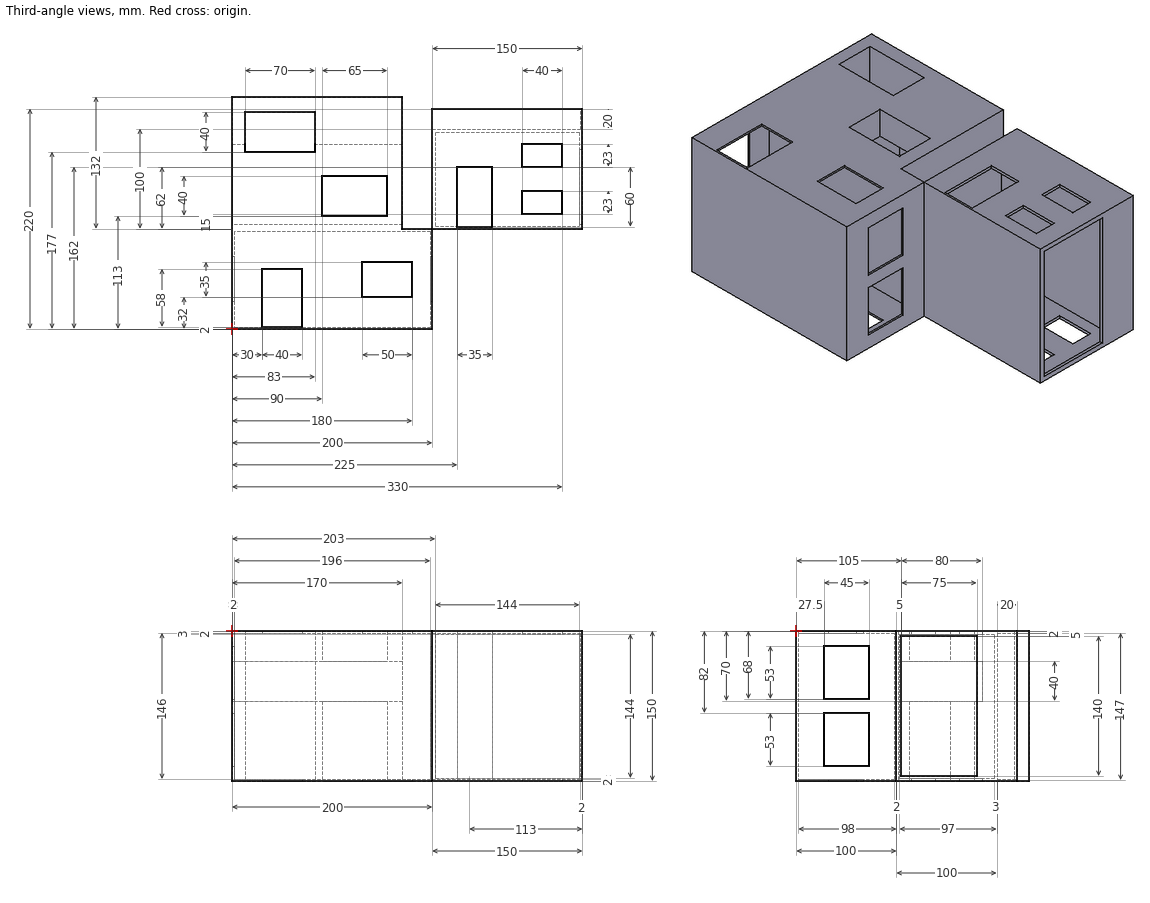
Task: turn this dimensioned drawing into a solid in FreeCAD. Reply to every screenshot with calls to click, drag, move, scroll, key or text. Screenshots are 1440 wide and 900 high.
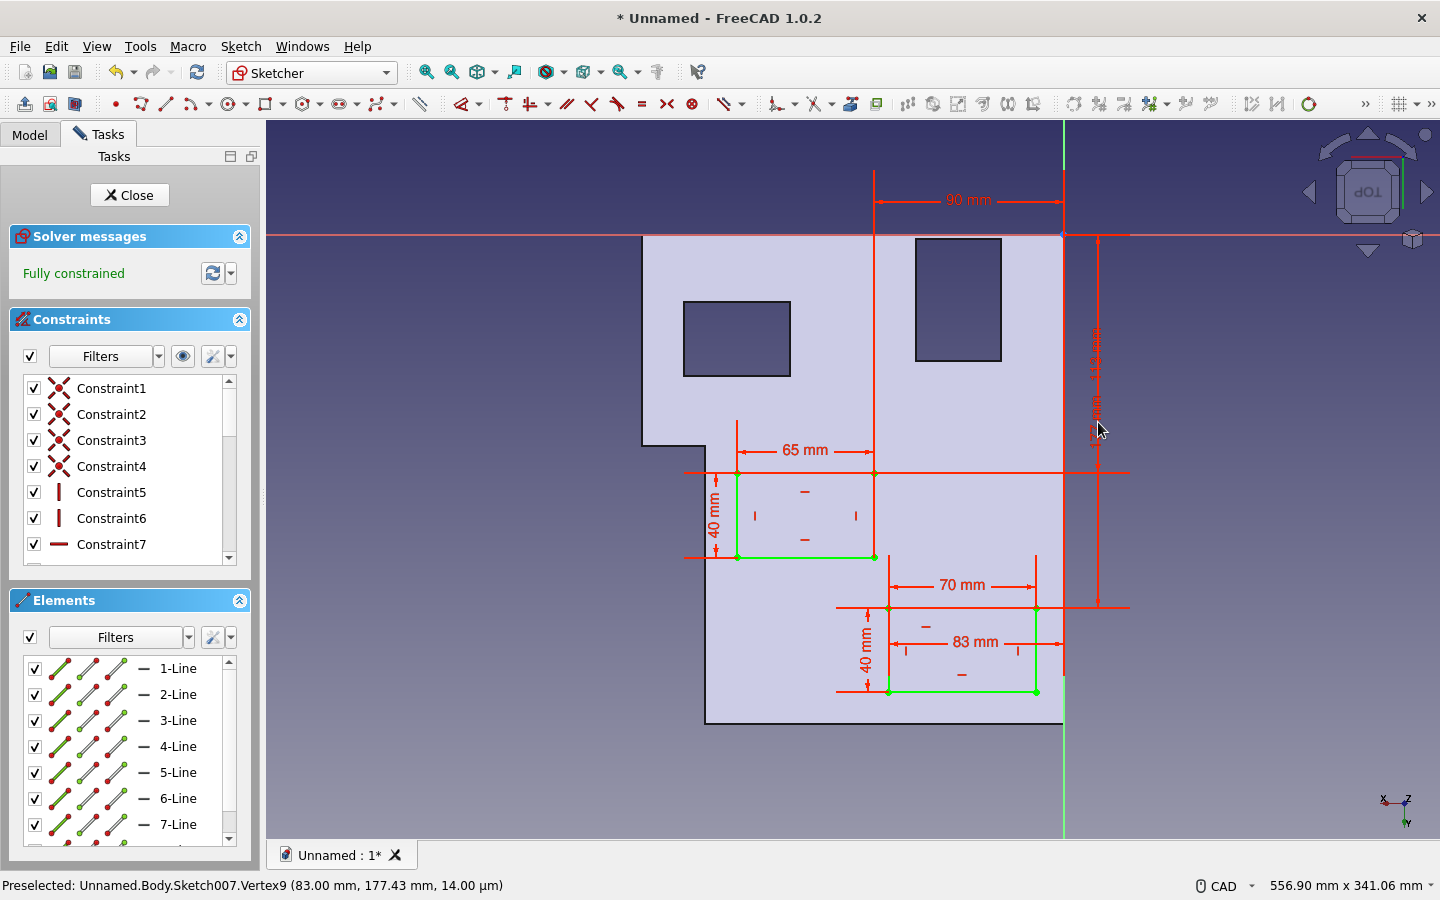
click(130, 195)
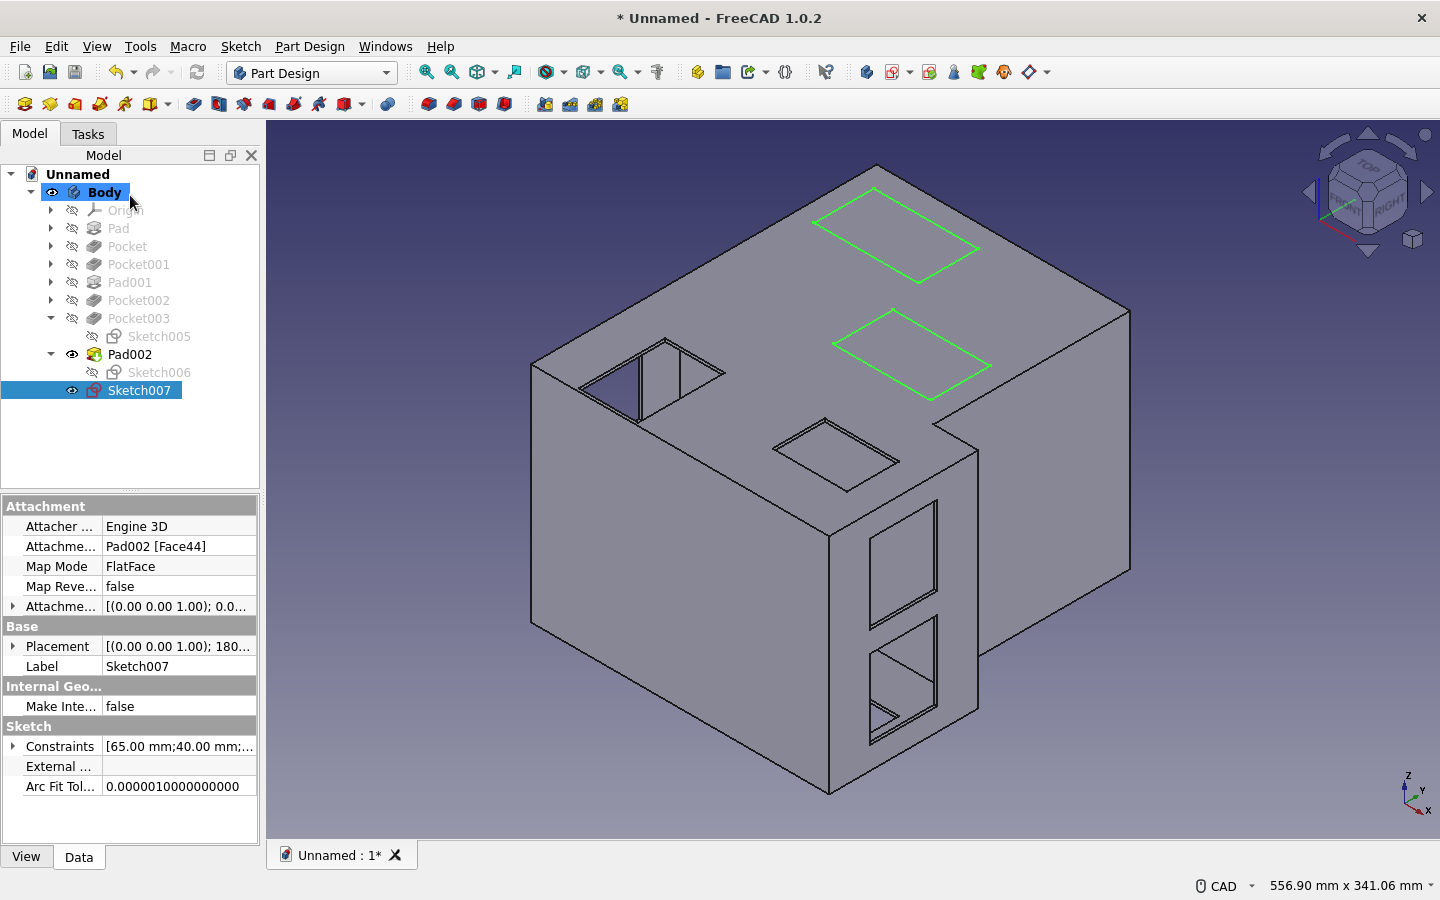
click(194, 104)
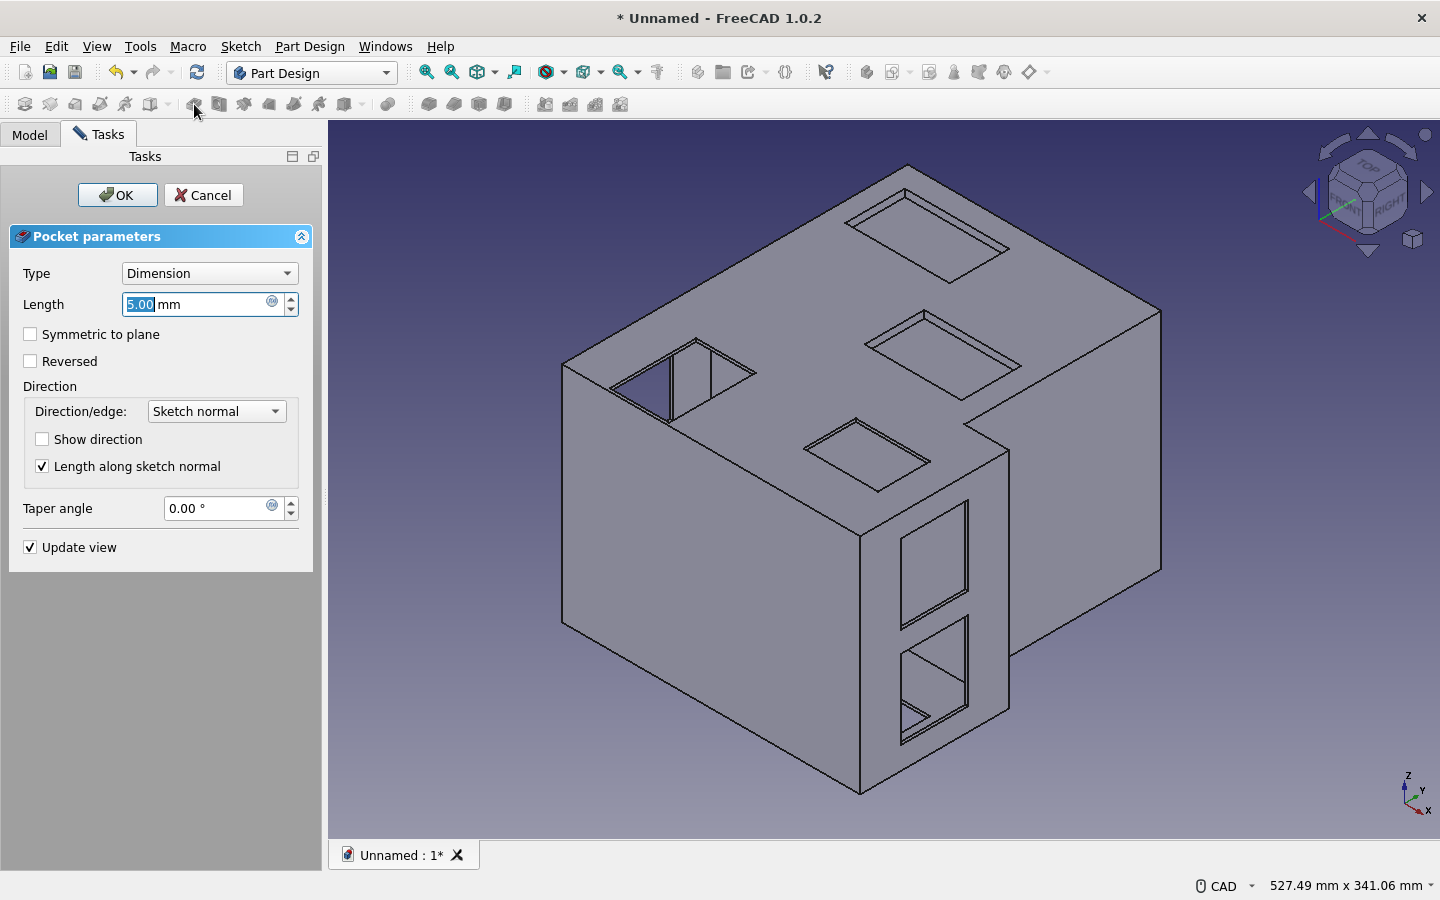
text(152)
key(Tab)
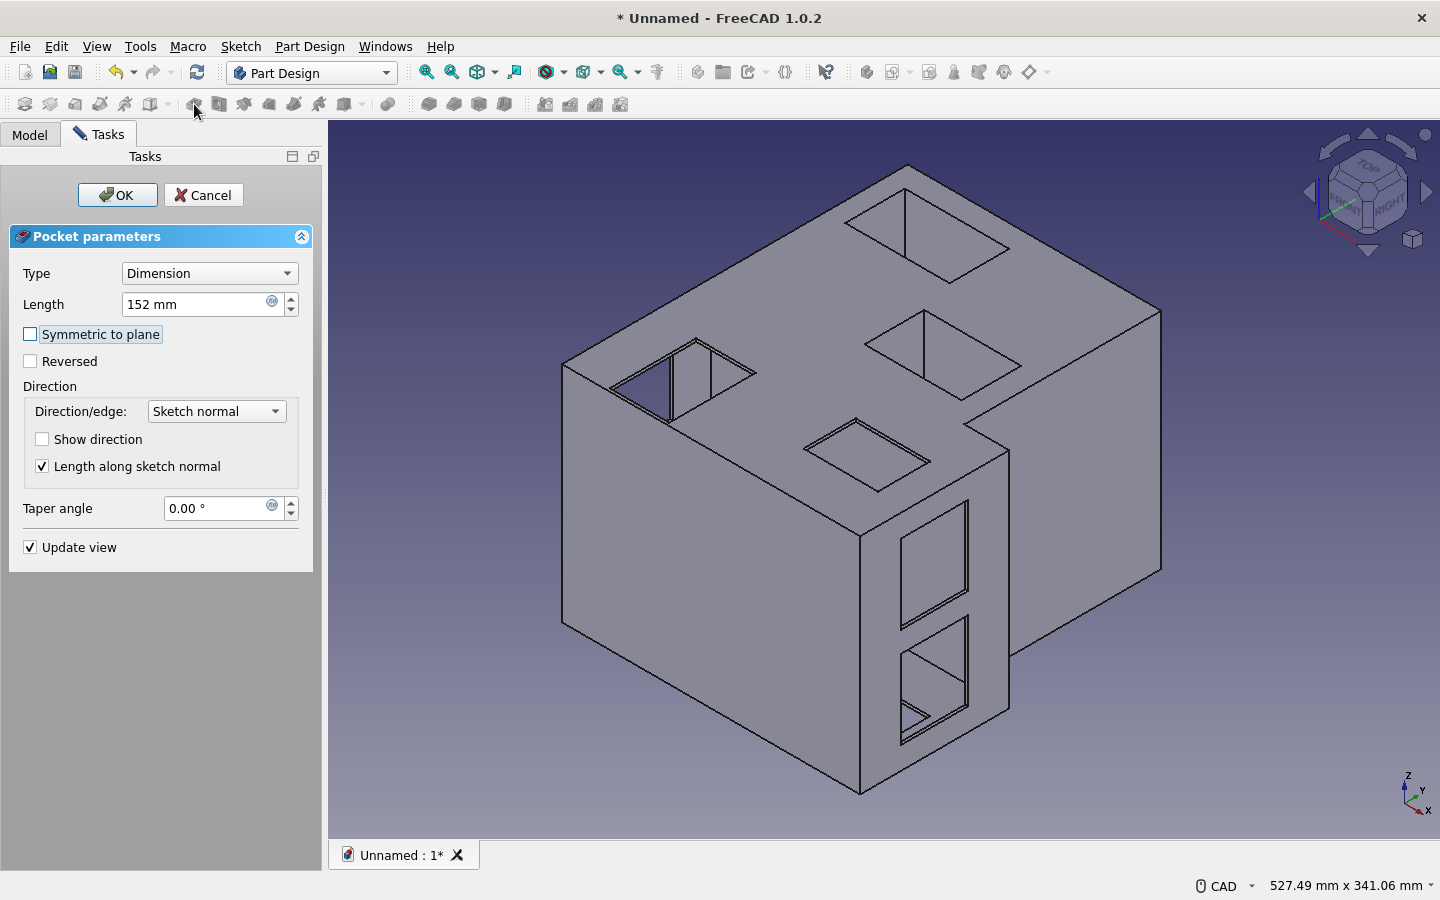
click(118, 195)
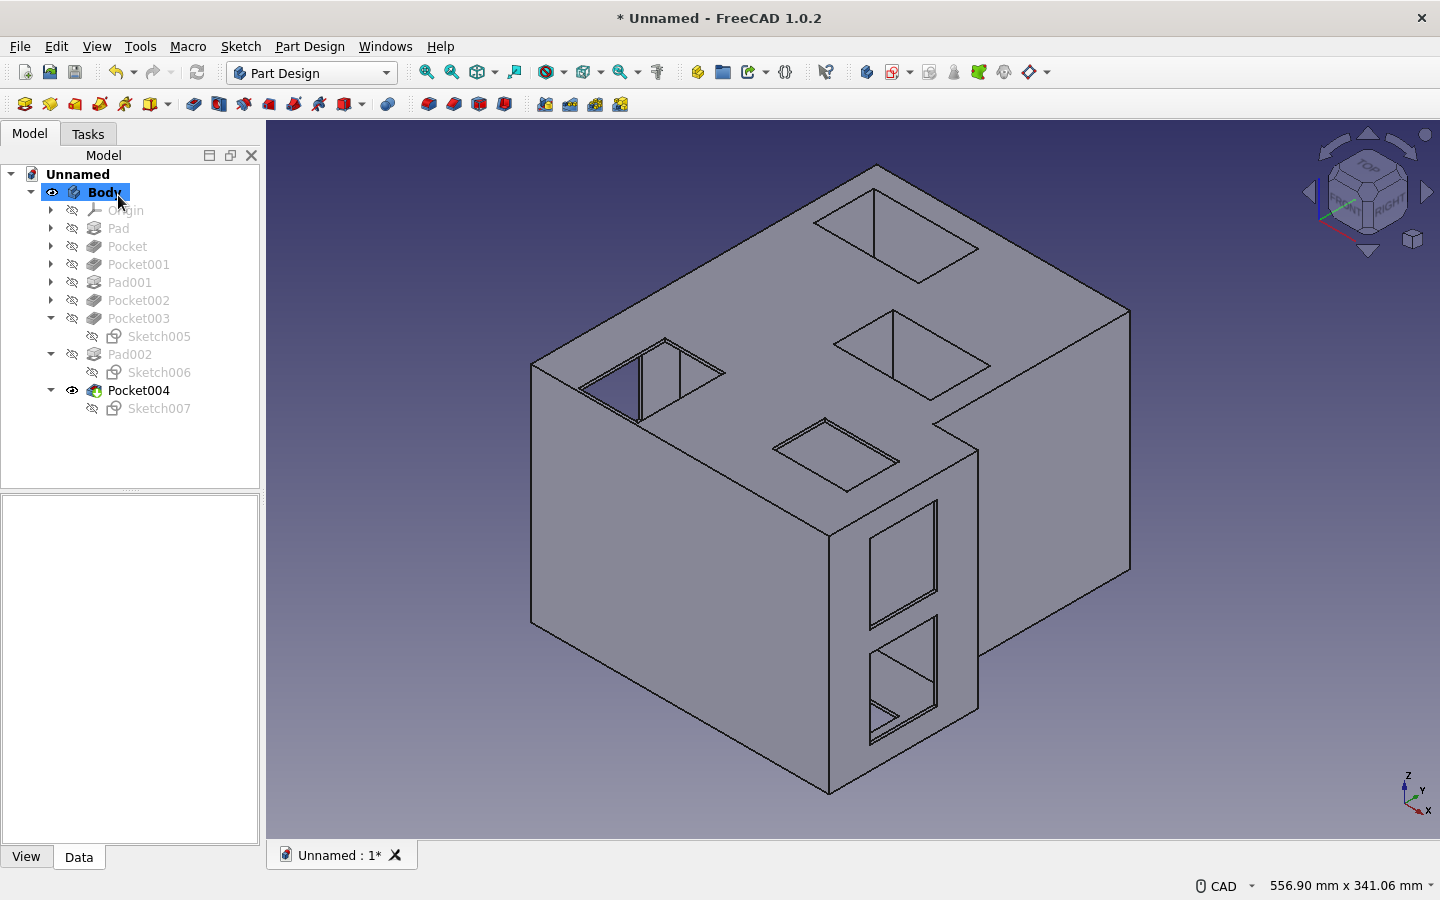
click(1032, 496)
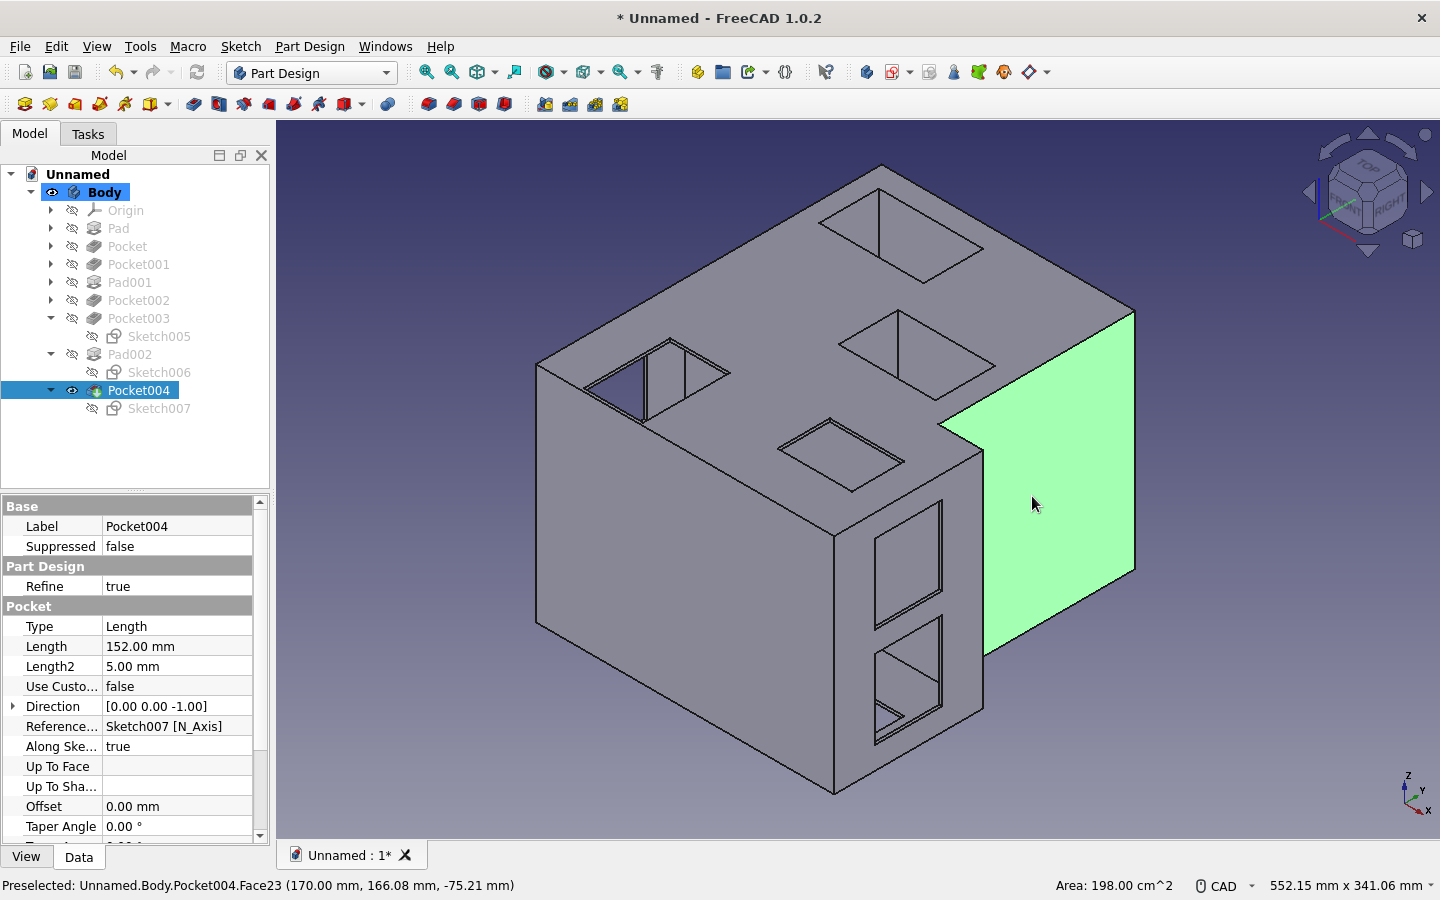
click(892, 72)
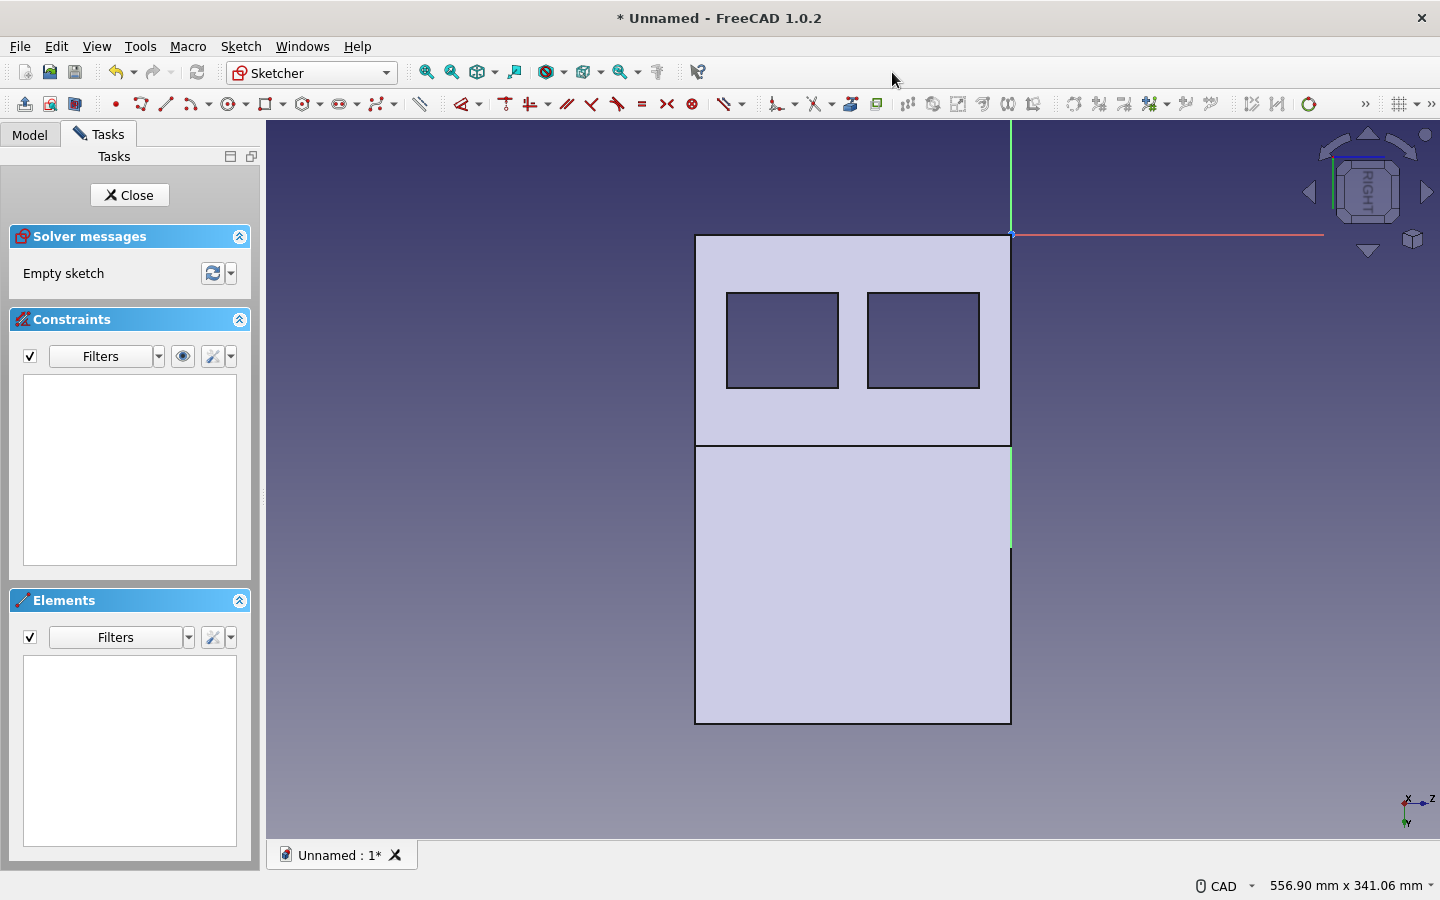
click(264, 104)